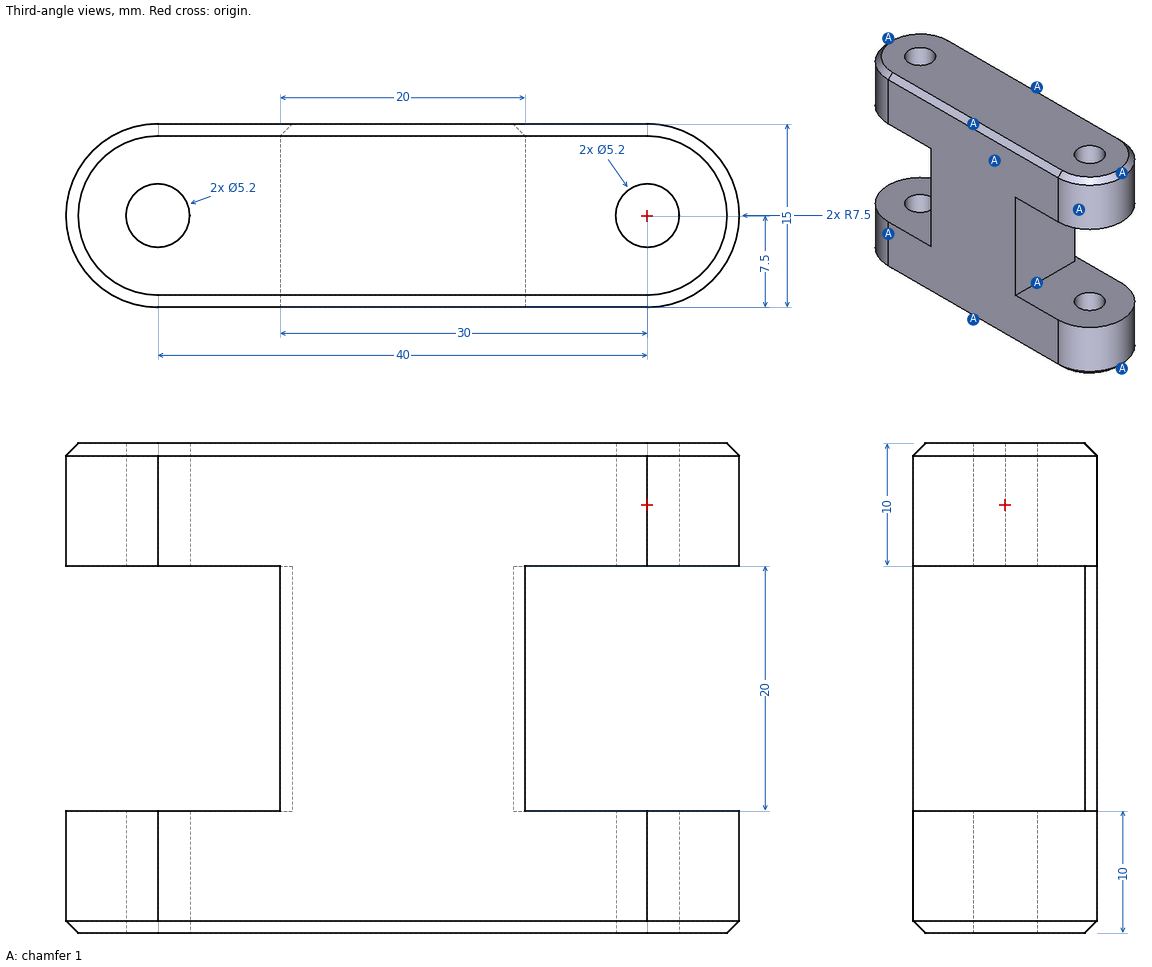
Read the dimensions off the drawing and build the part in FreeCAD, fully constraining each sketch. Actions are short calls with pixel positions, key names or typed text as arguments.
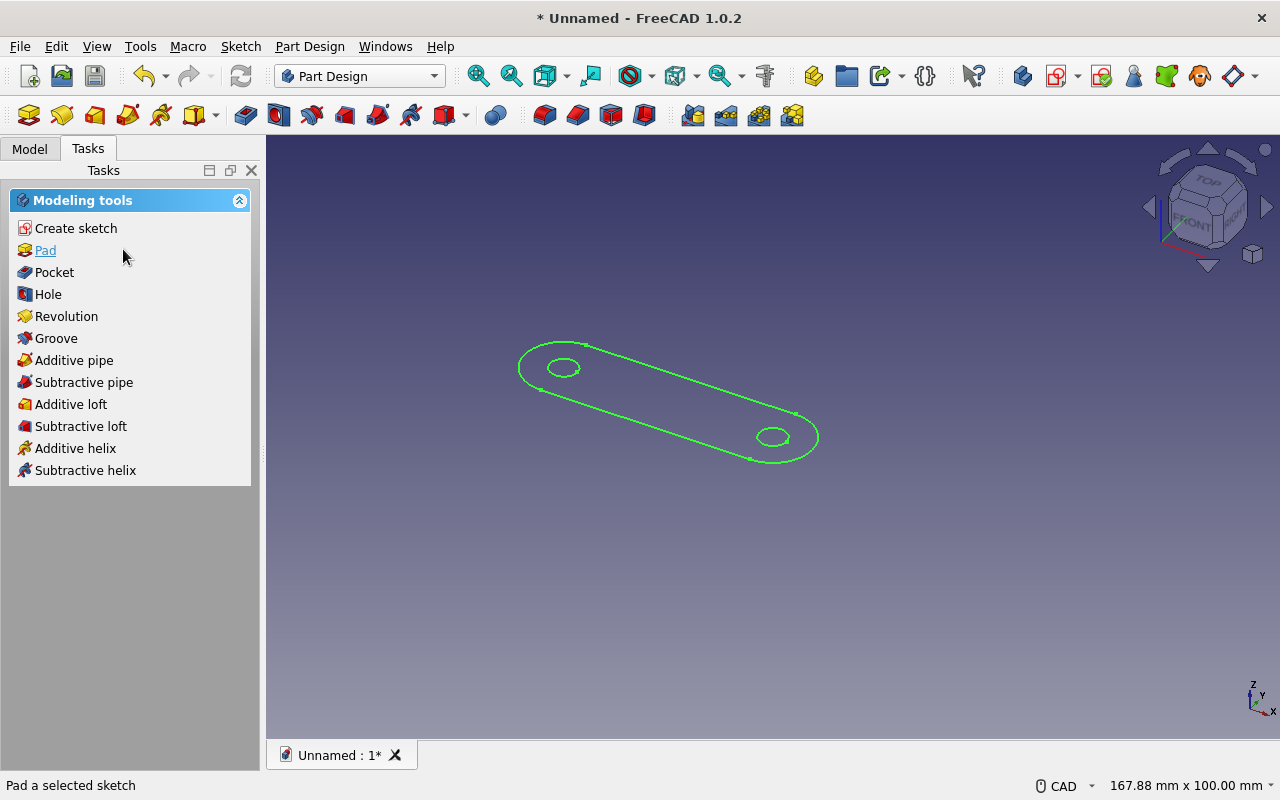
click(29, 116)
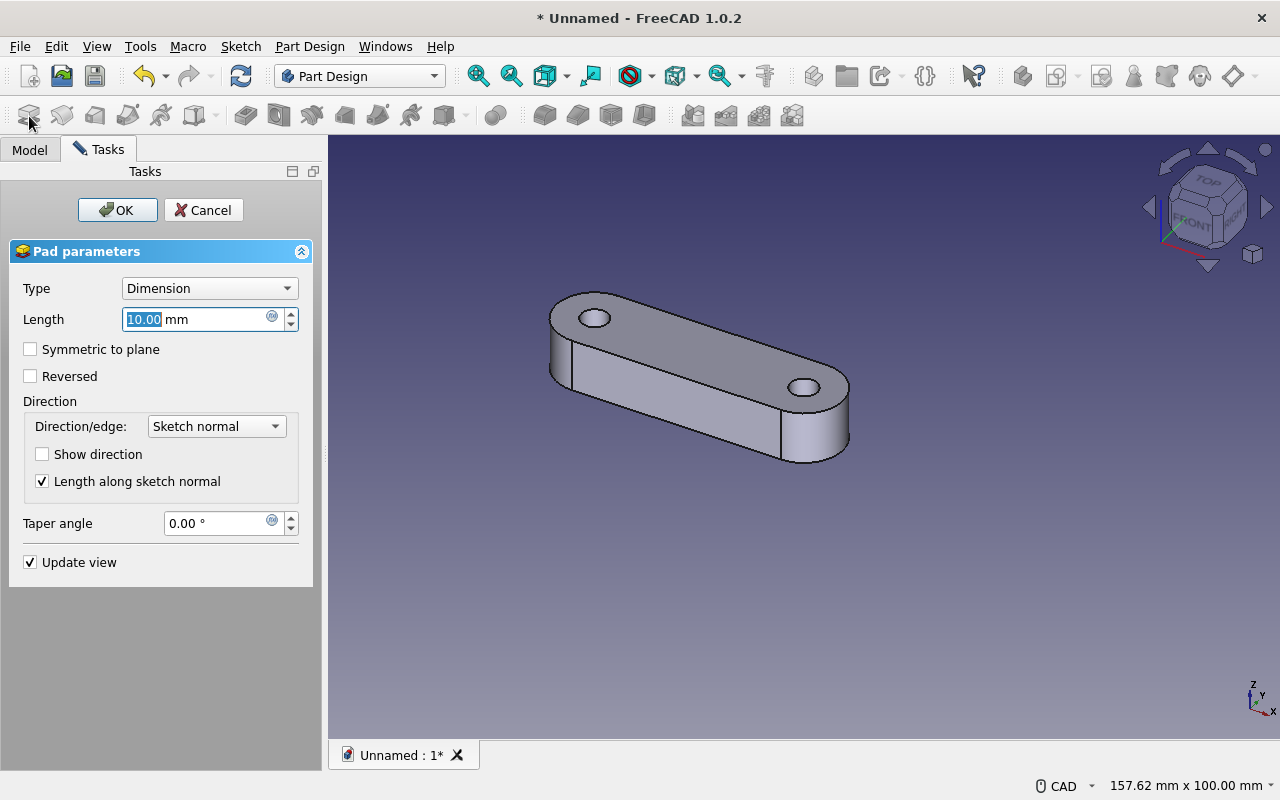
text(10)
key(Tab)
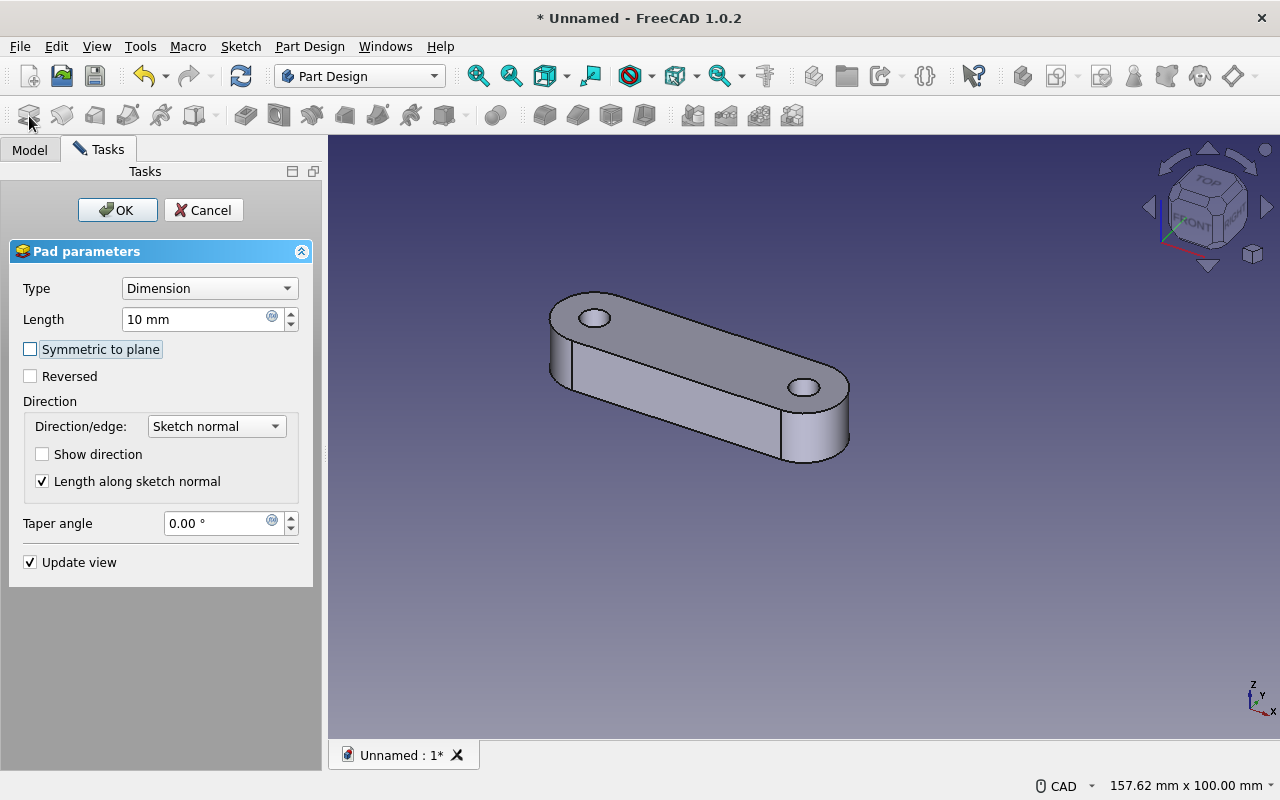
click(31, 349)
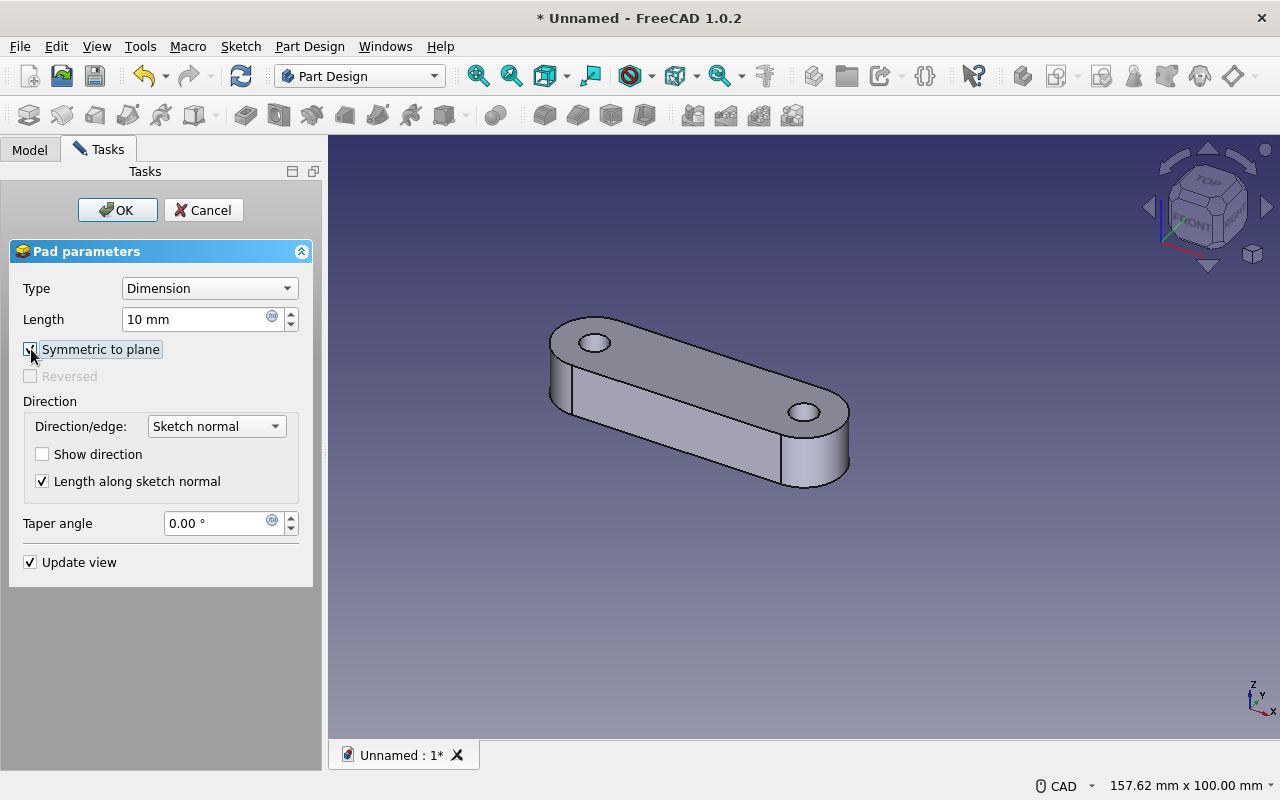
click(118, 210)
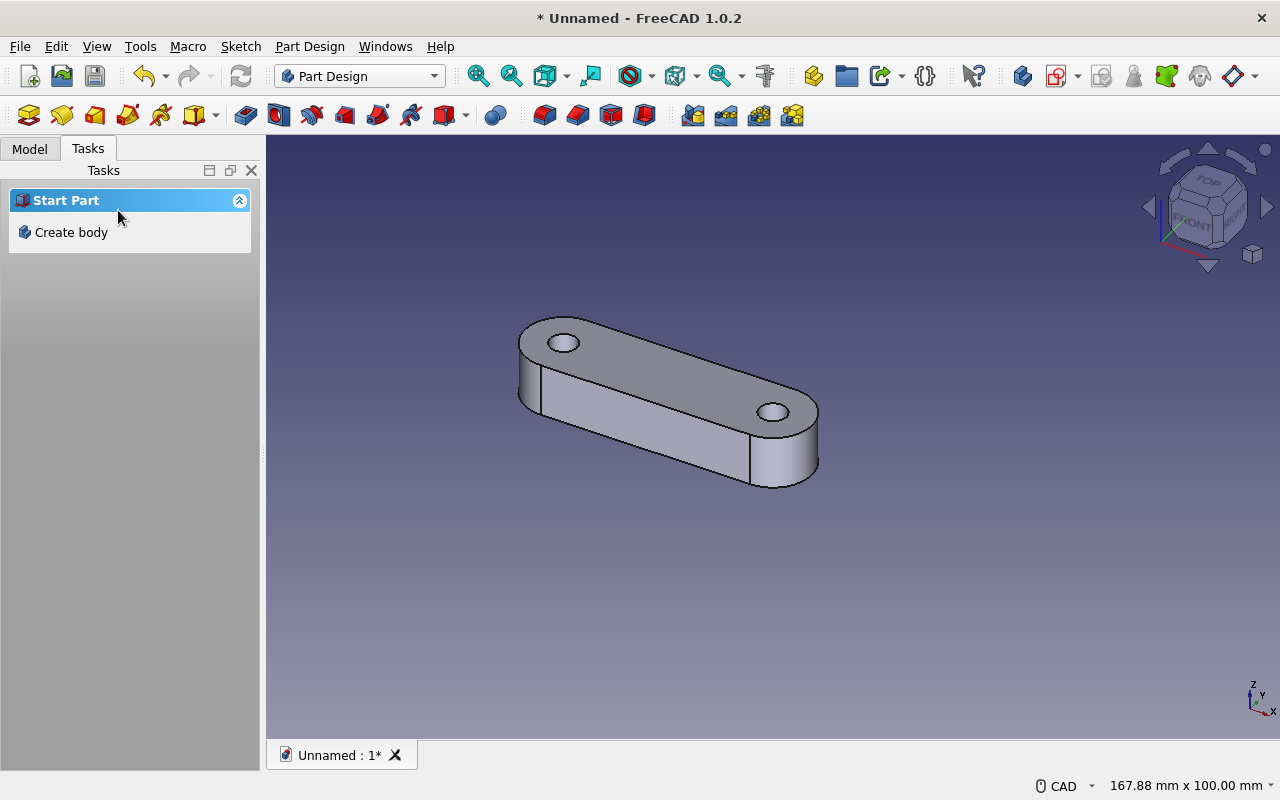
key(v)
key(f)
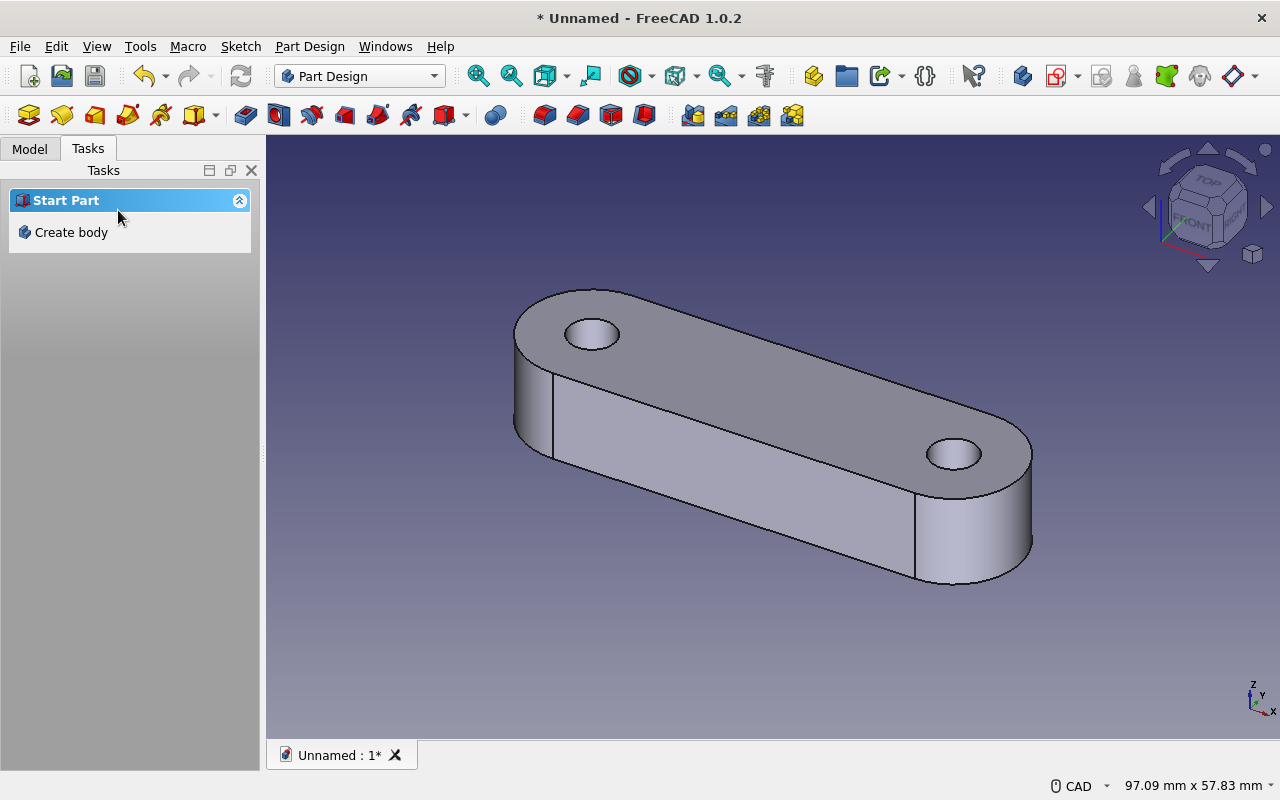
key(5)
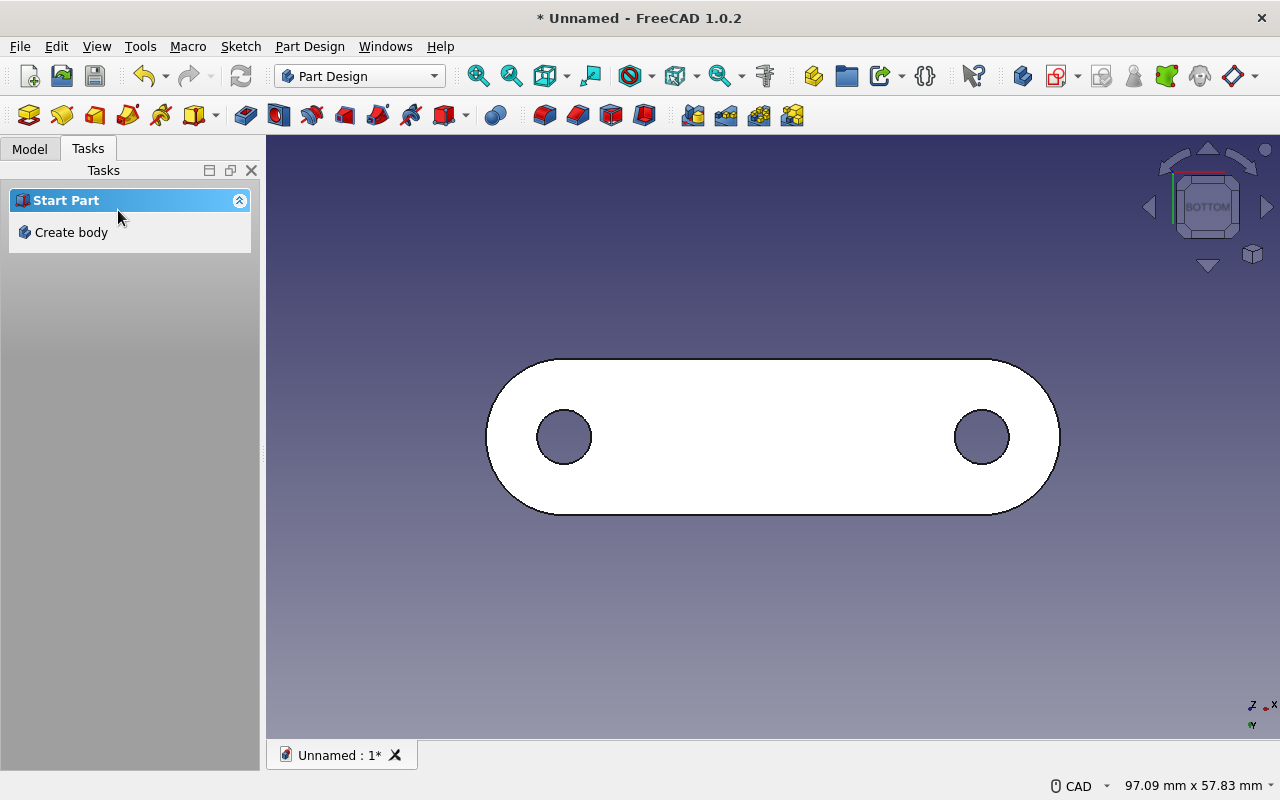
click(855, 436)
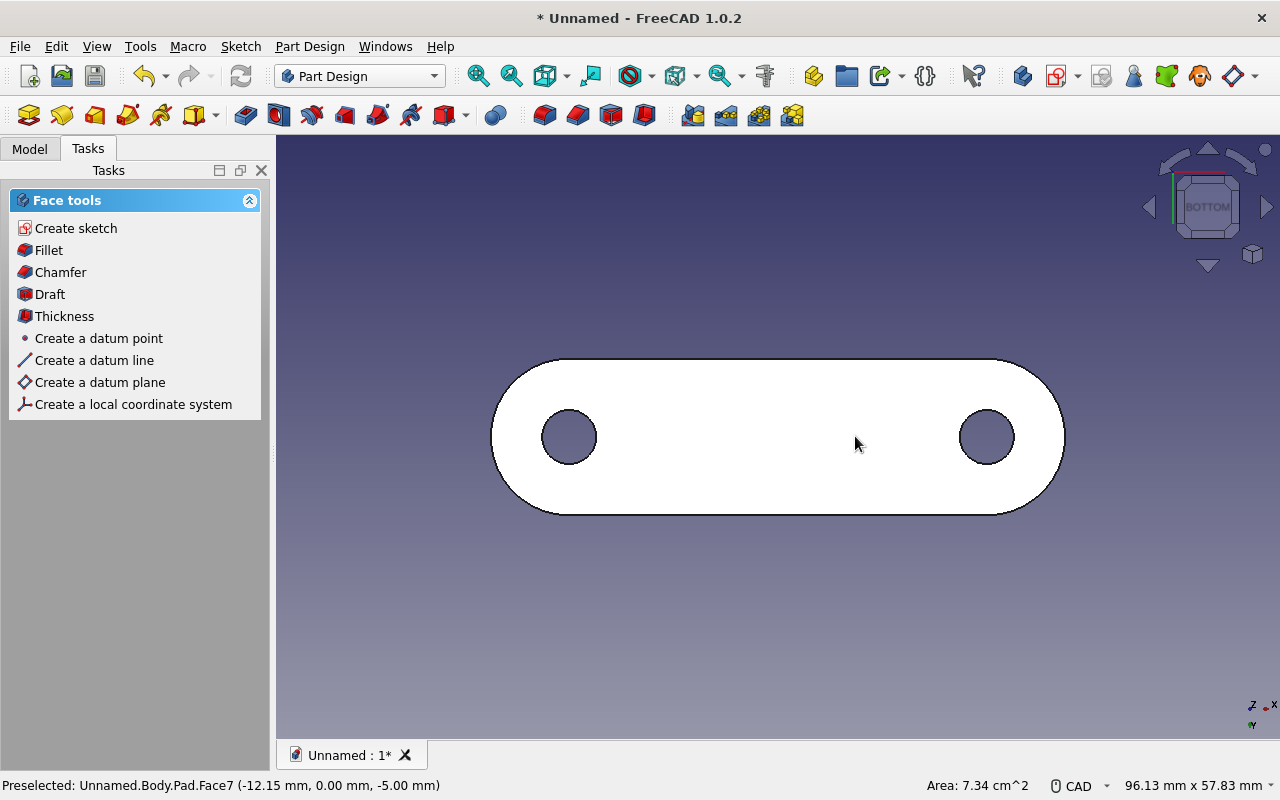
click(1056, 76)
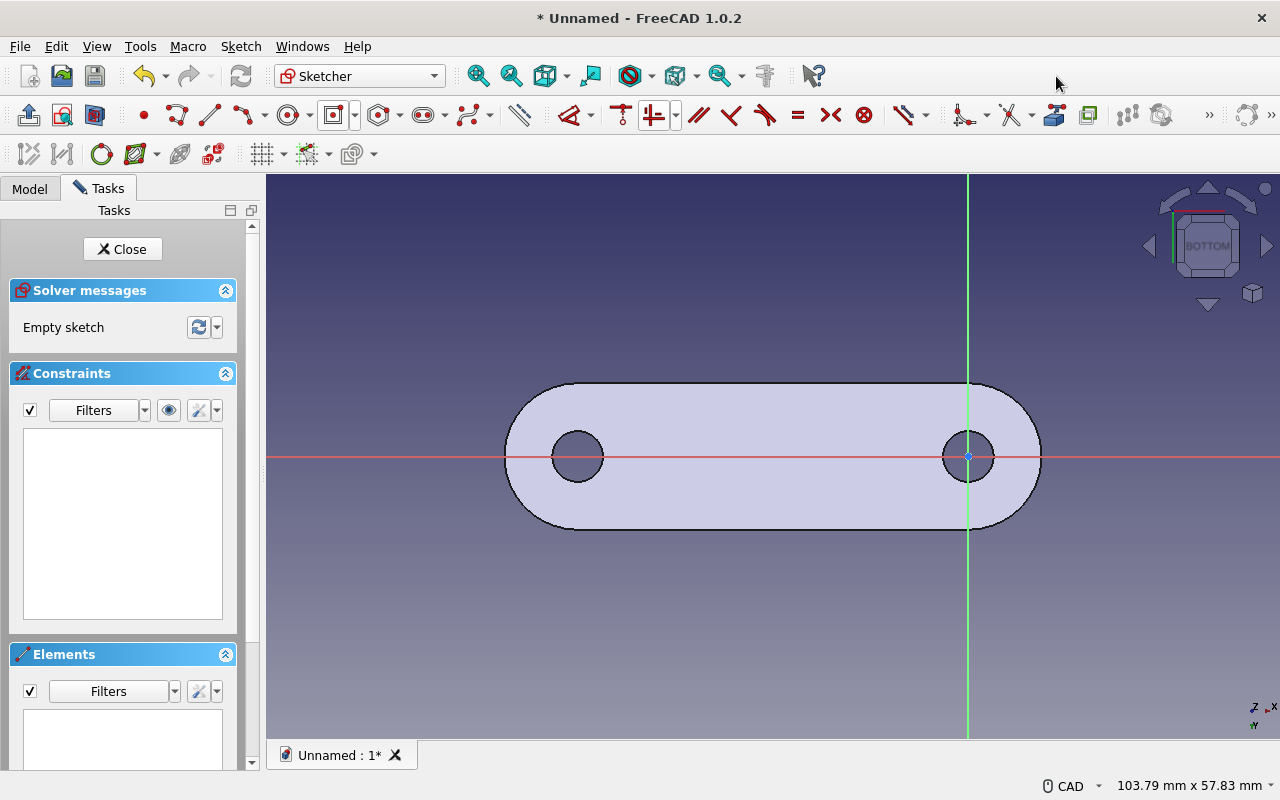
scroll(965, 456, up, 3)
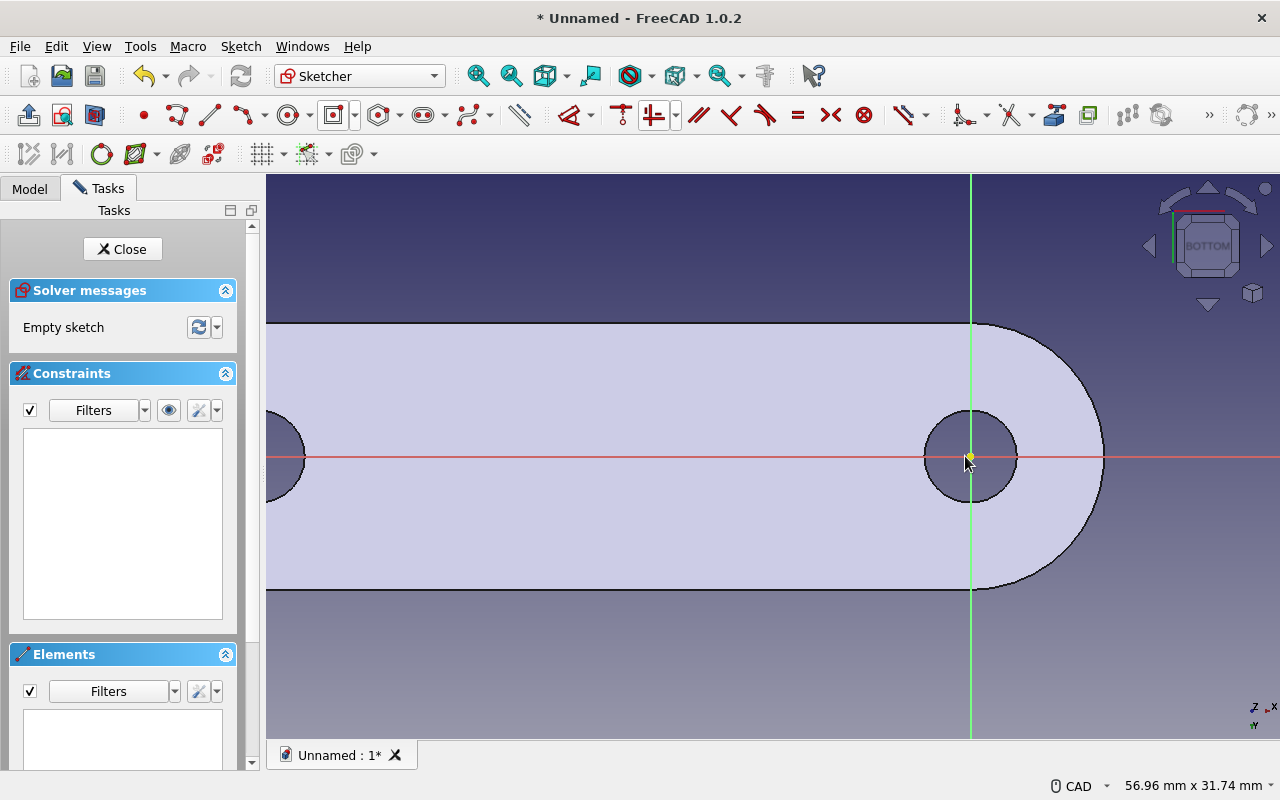
key(g)
key(r)